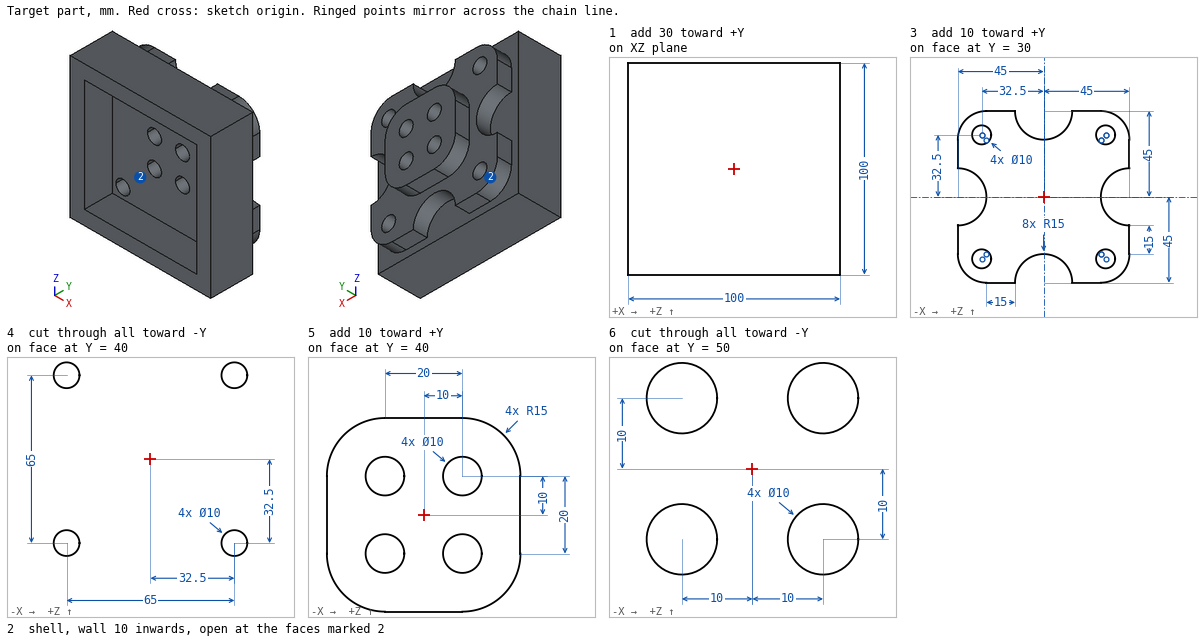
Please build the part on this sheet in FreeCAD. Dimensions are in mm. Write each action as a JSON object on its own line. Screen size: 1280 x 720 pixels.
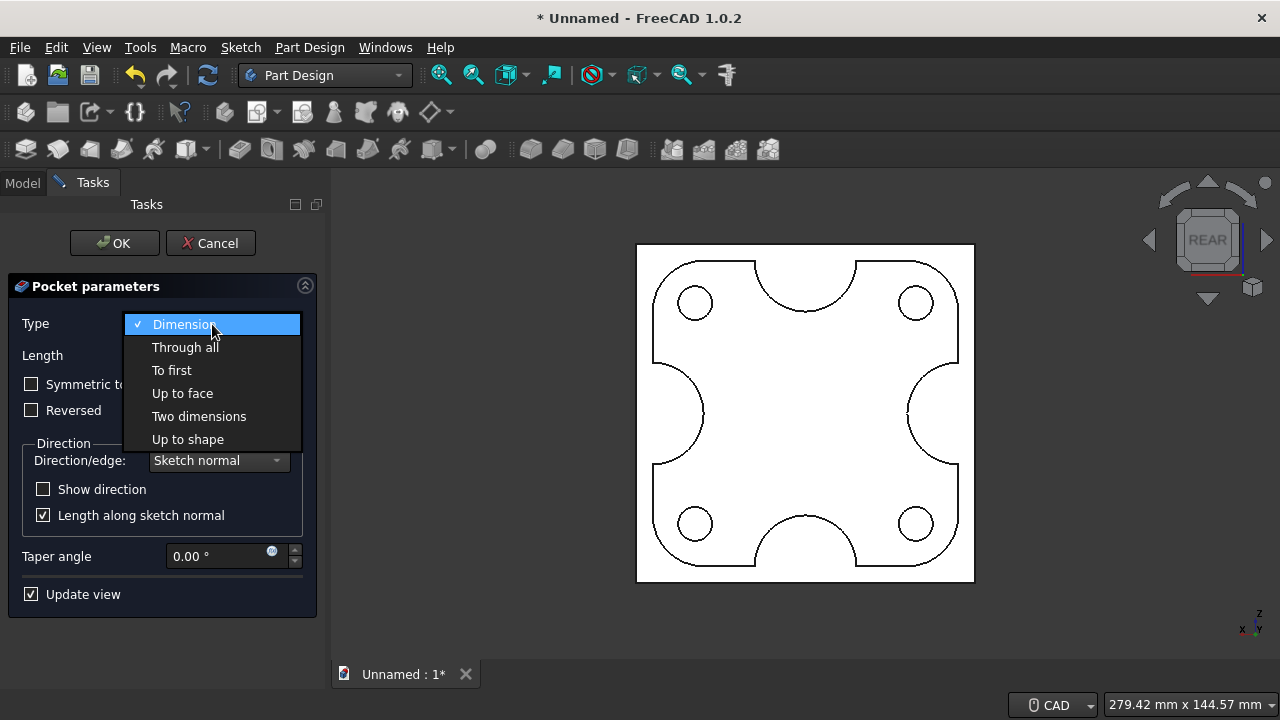
{"action": "left_click", "coordinate": [212, 348]}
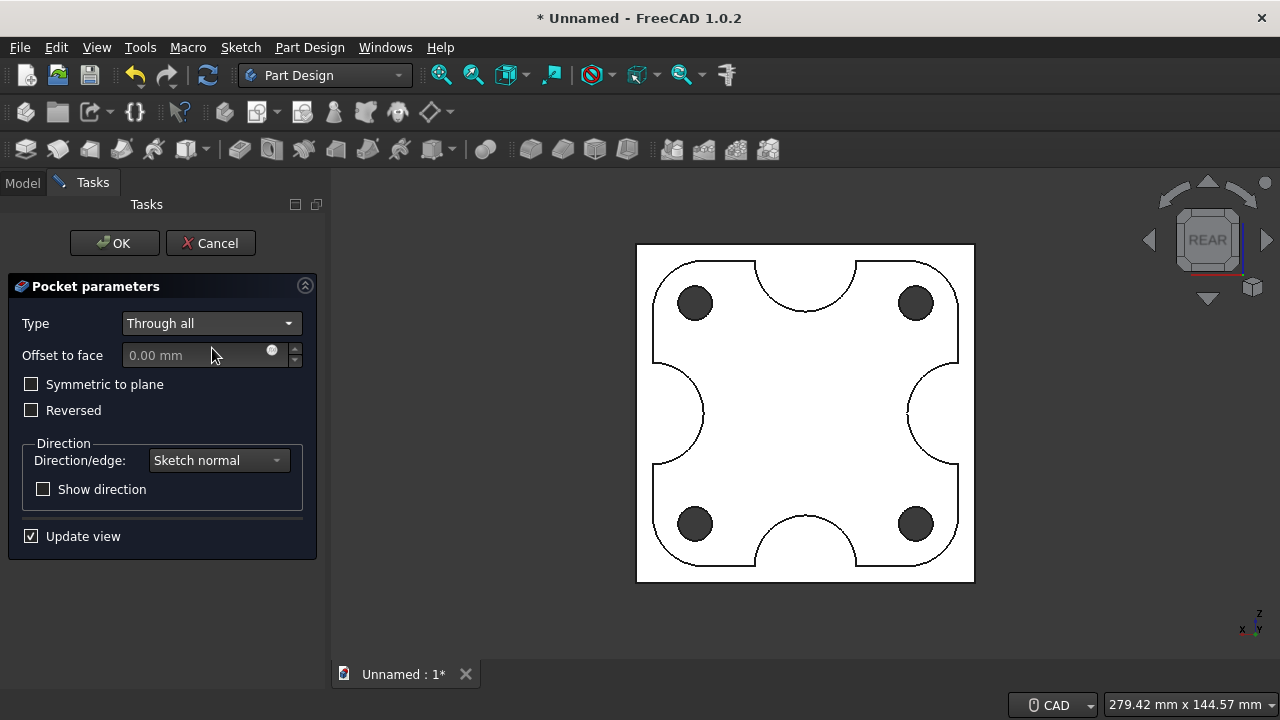
{"action": "left_click", "coordinate": [115, 243]}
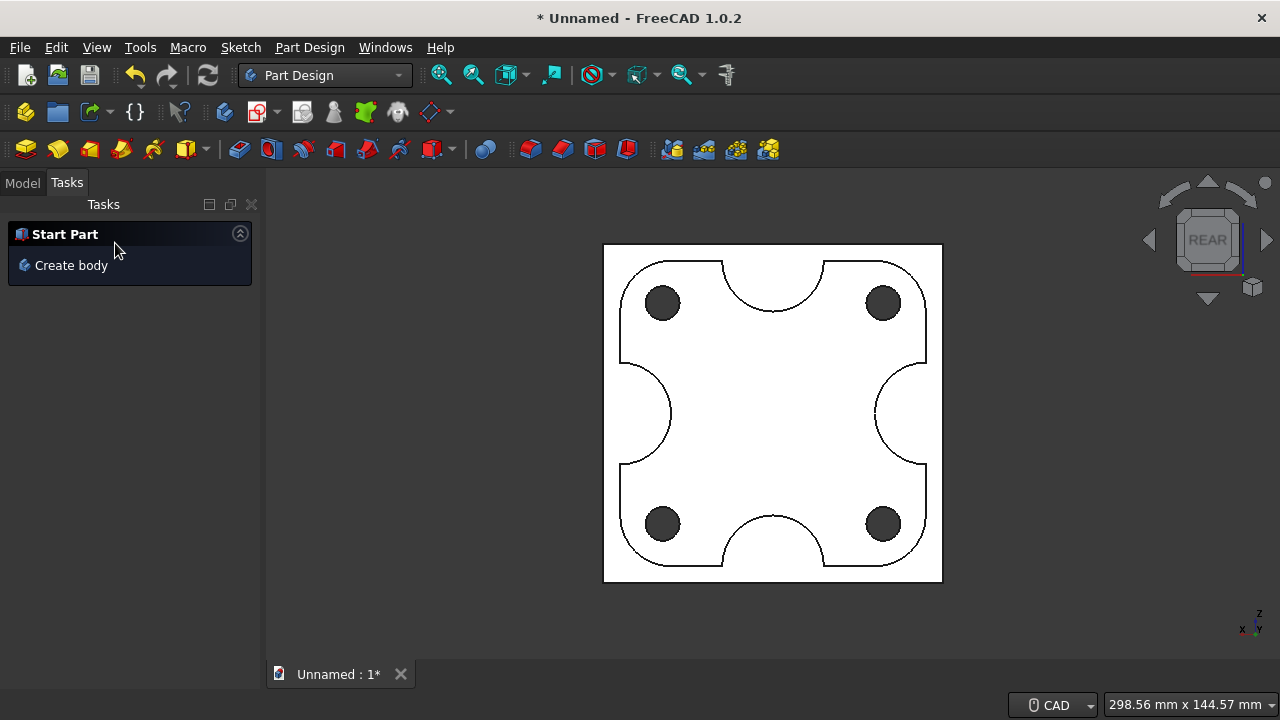
{"action": "left_click", "coordinate": [773, 412]}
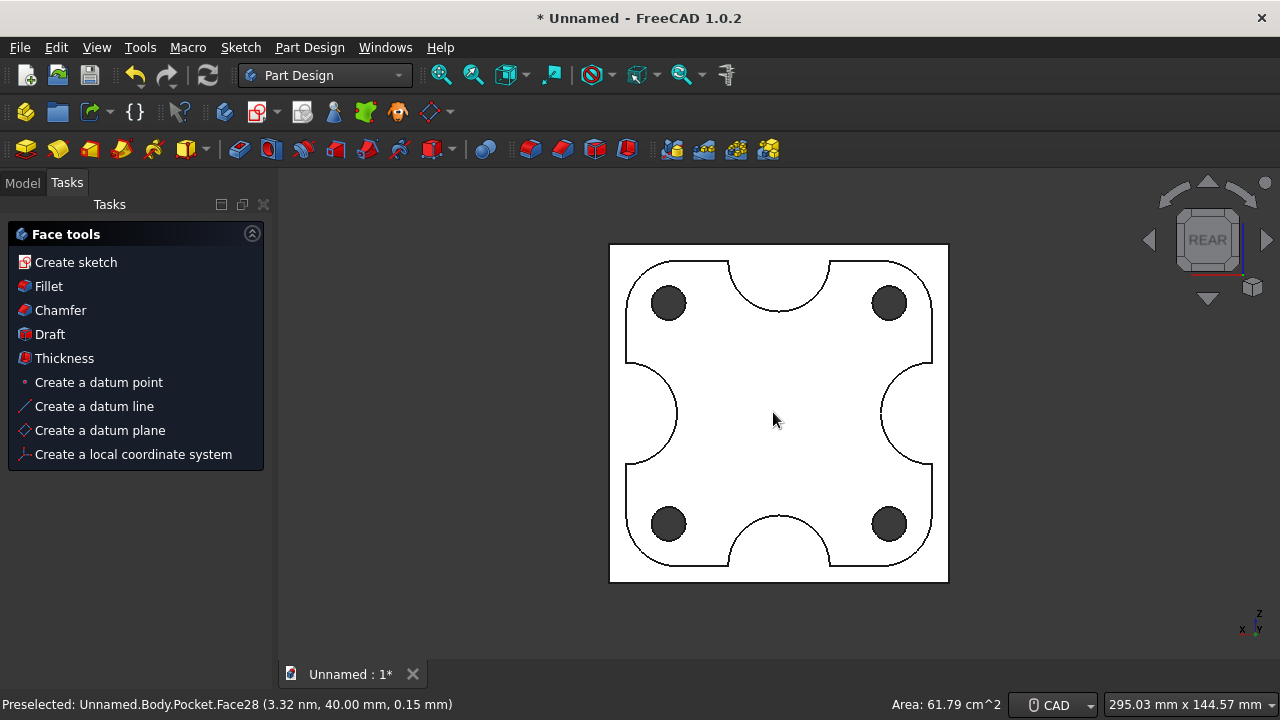
{"action": "left_click", "coordinate": [258, 112]}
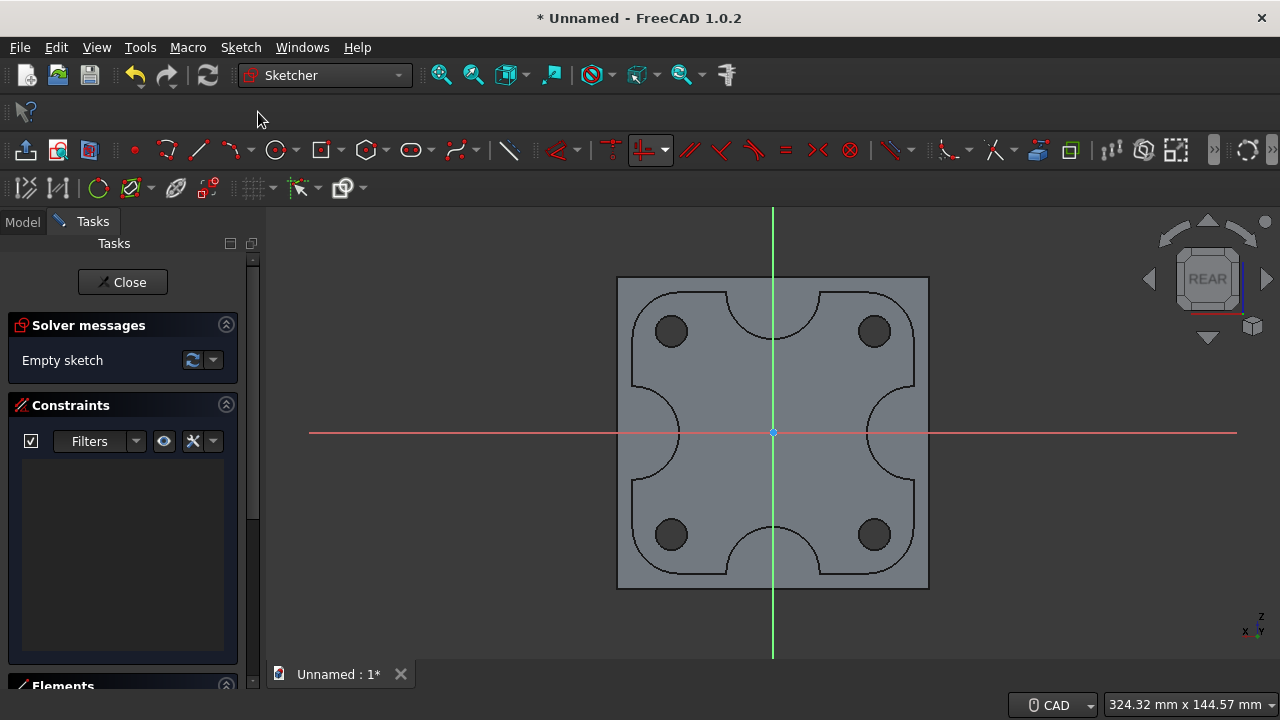
{"action": "scroll", "coordinate": [856, 433], "scroll_direction": "up", "scroll_amount": 3}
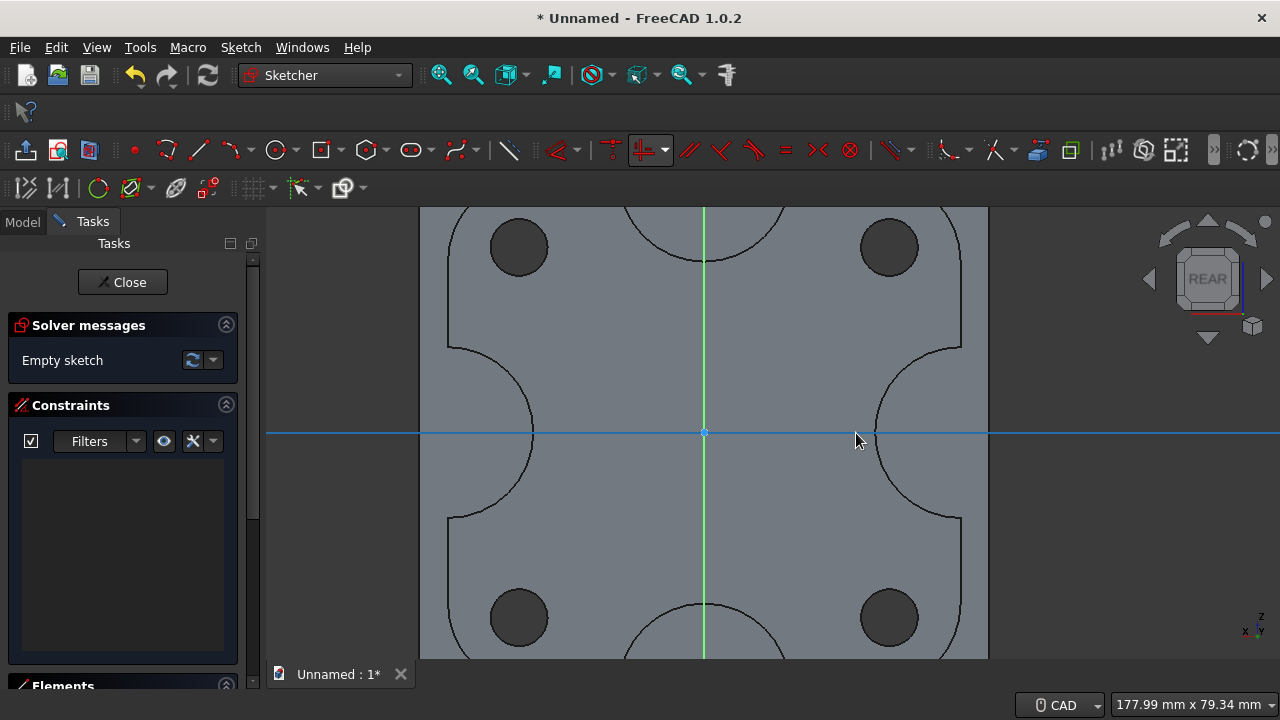
{"action": "left_click", "coordinate": [200, 150]}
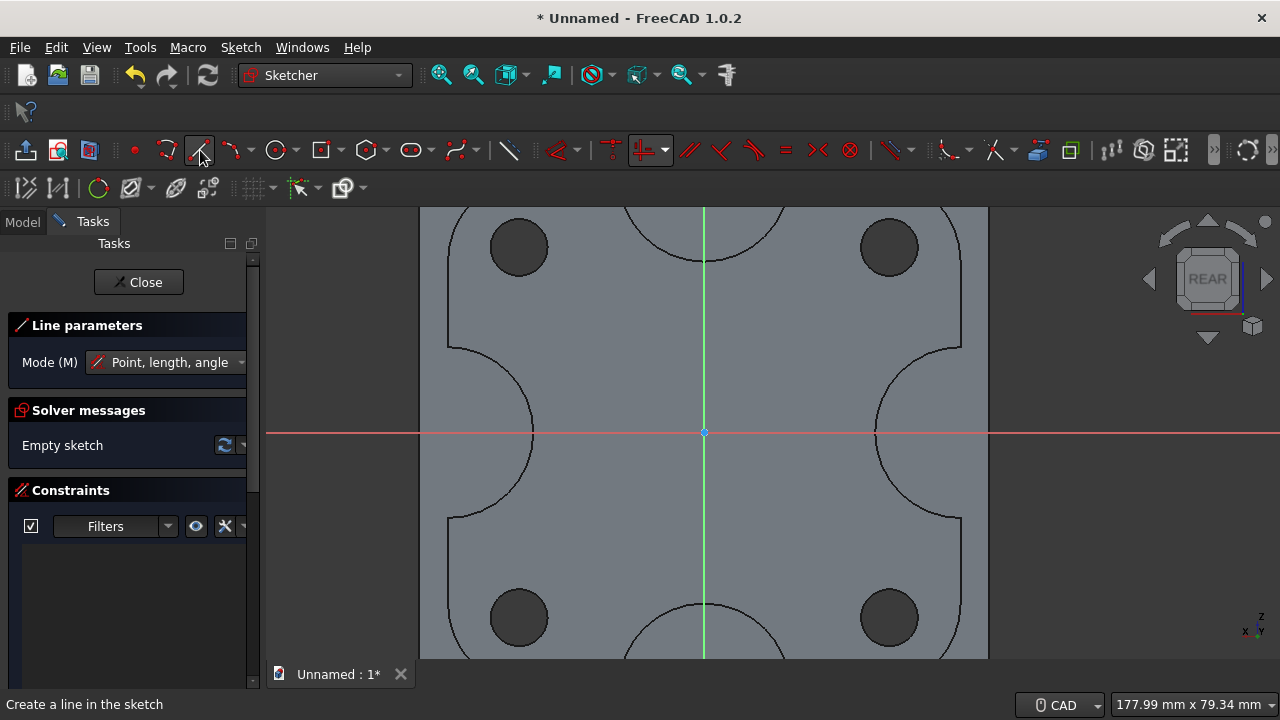
{"action": "left_click", "coordinate": [847, 490]}
{"action": "left_click", "coordinate": [847, 376]}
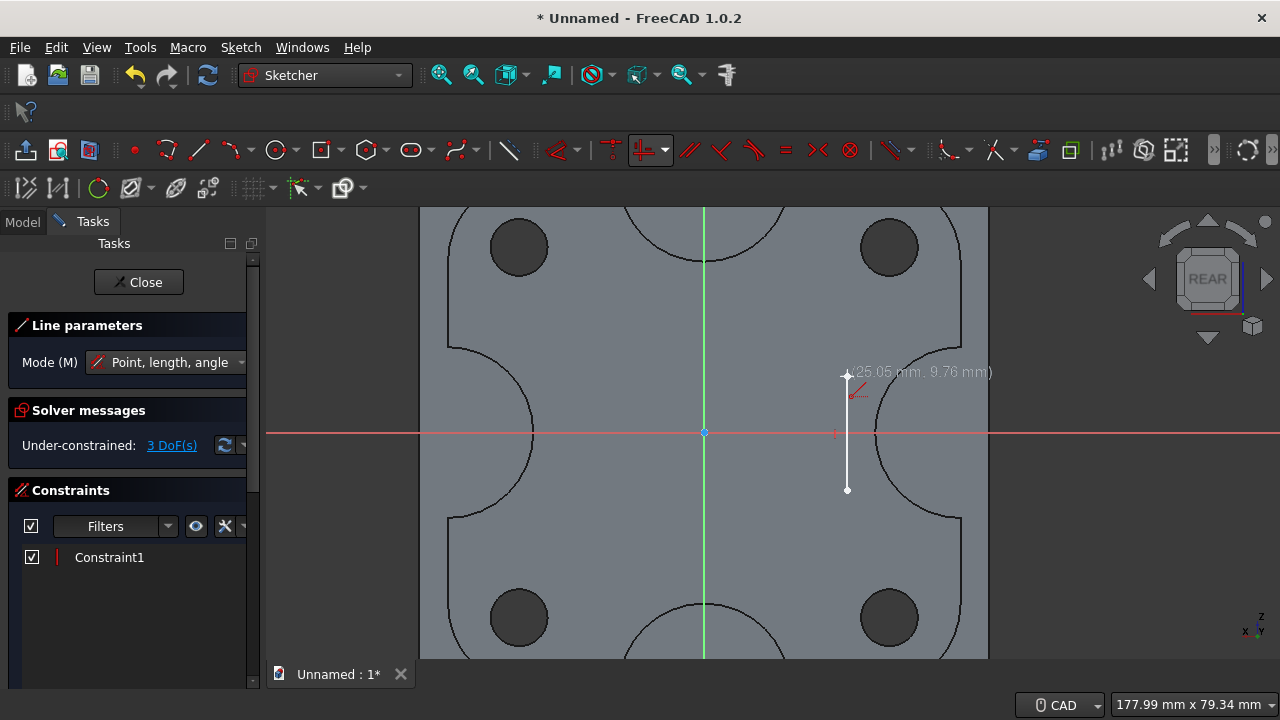
{"action": "left_click", "coordinate": [761, 290]}
{"action": "left_click", "coordinate": [647, 290]}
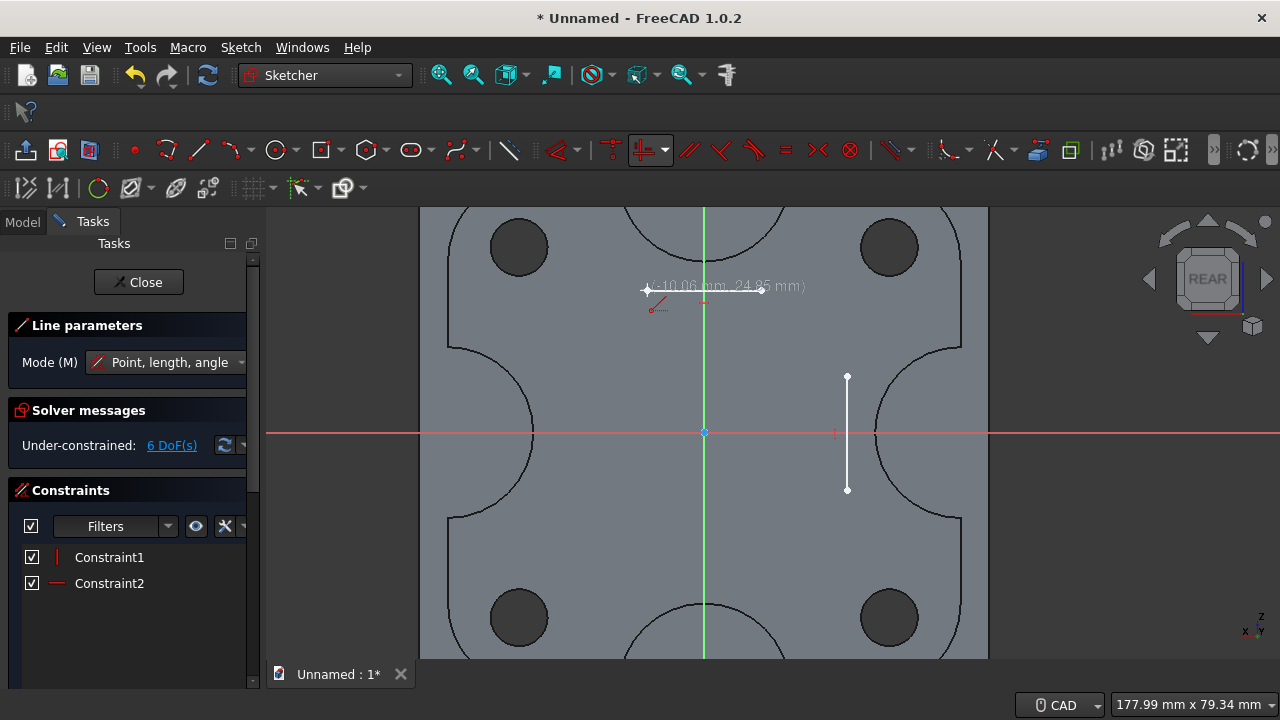
{"action": "left_click", "coordinate": [562, 376]}
{"action": "left_click", "coordinate": [562, 490]}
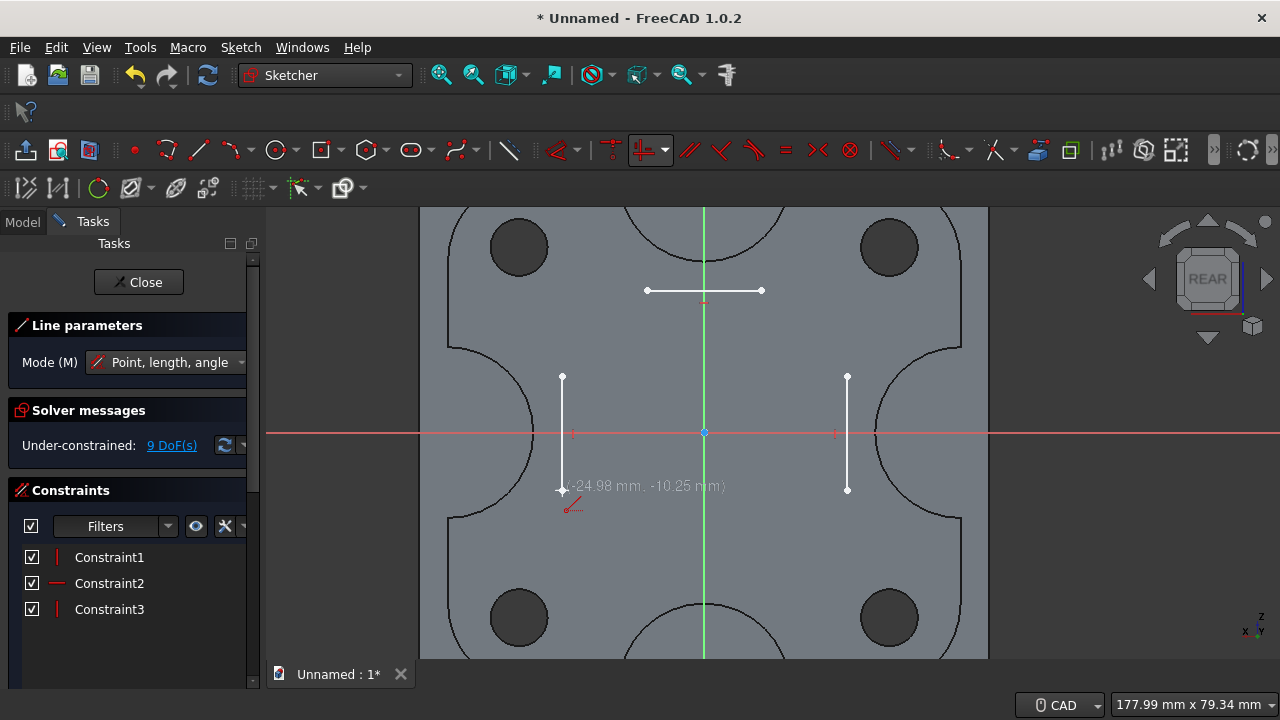
{"action": "left_click", "coordinate": [647, 575]}
{"action": "left_click", "coordinate": [761, 575]}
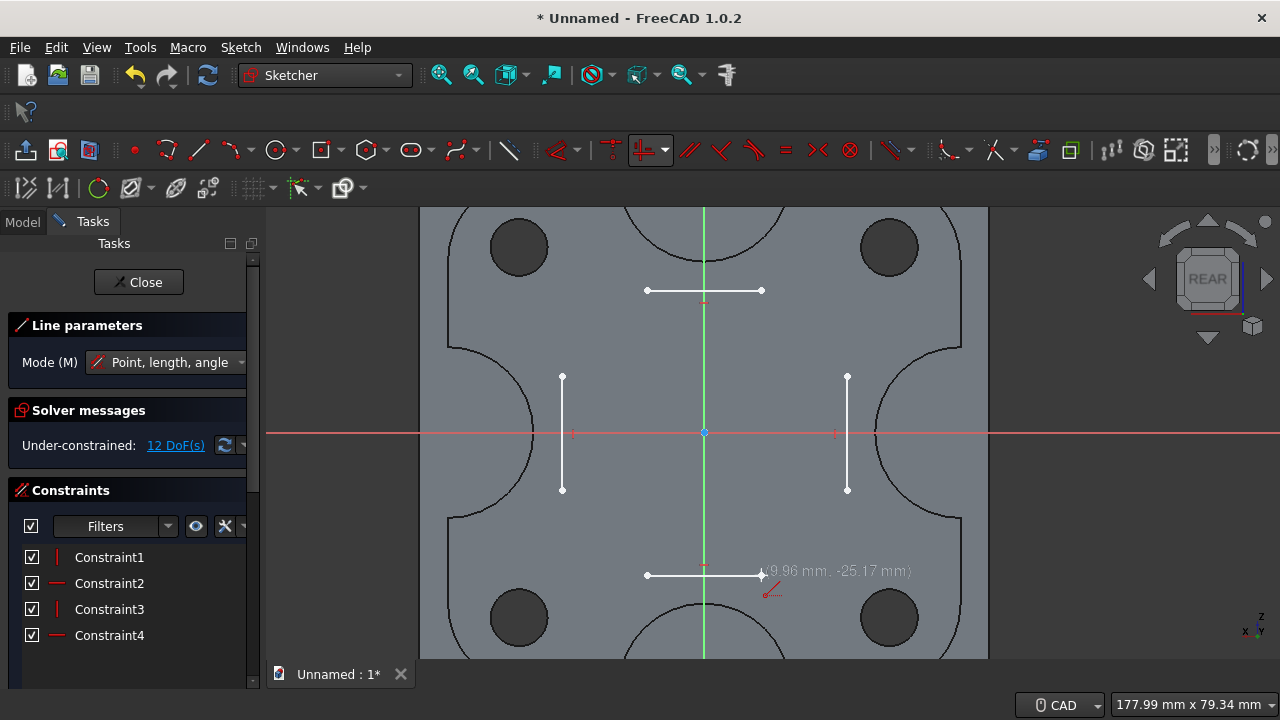
{"action": "left_click", "coordinate": [232, 150]}